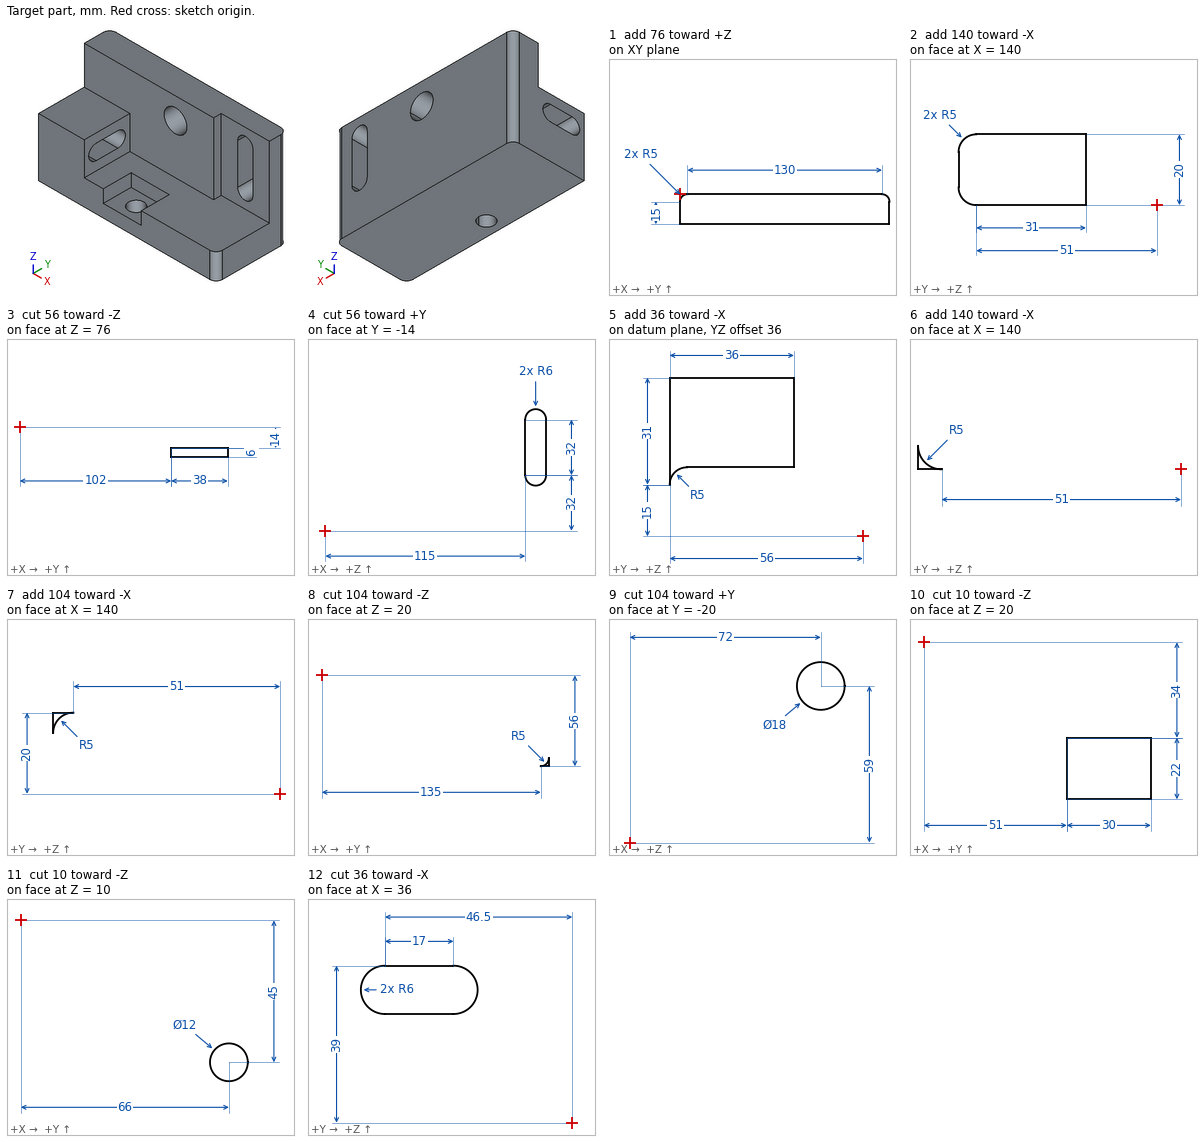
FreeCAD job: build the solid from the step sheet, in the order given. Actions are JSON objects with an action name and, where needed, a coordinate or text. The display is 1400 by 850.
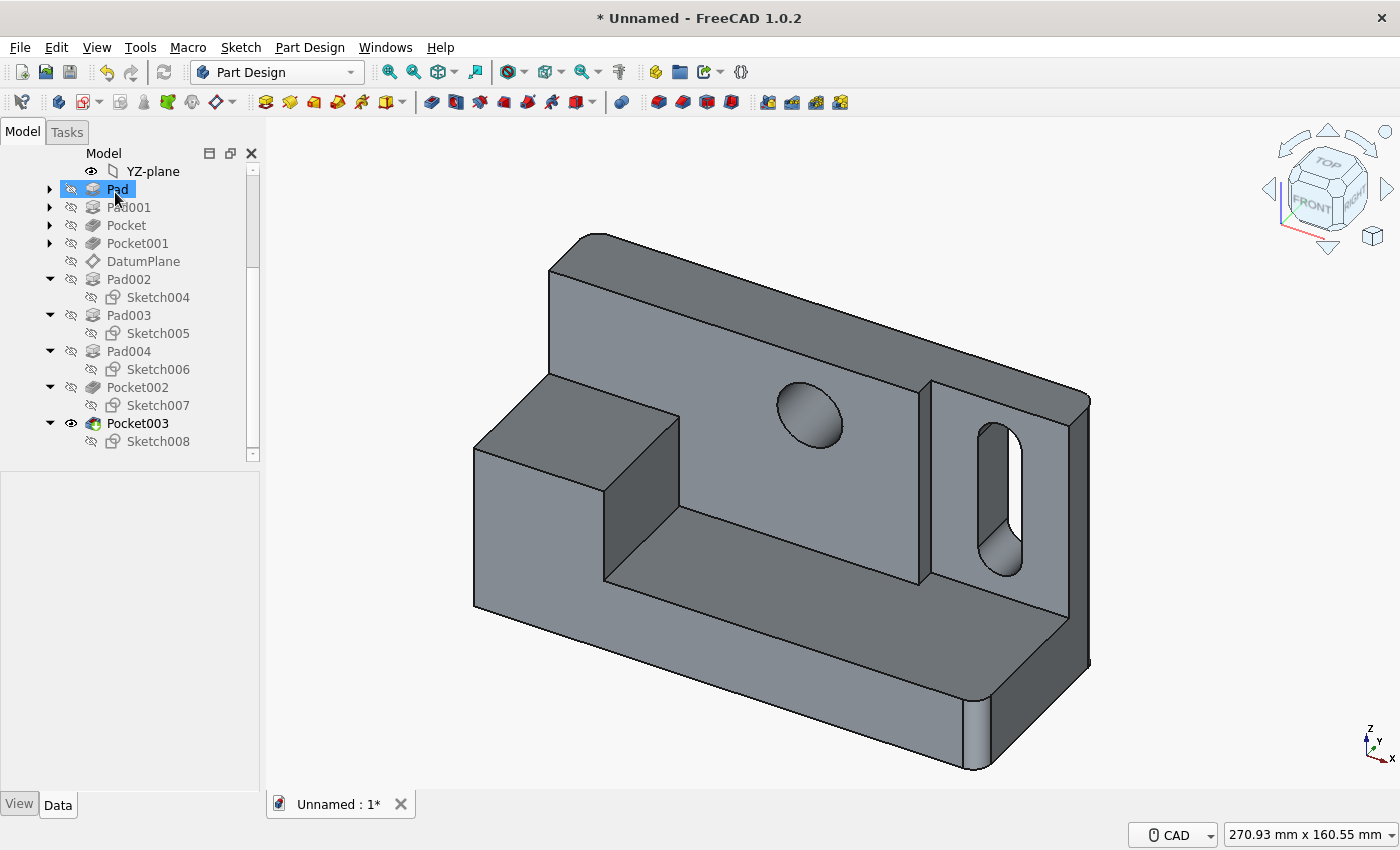
{"action": "left_click", "coordinate": [944, 634]}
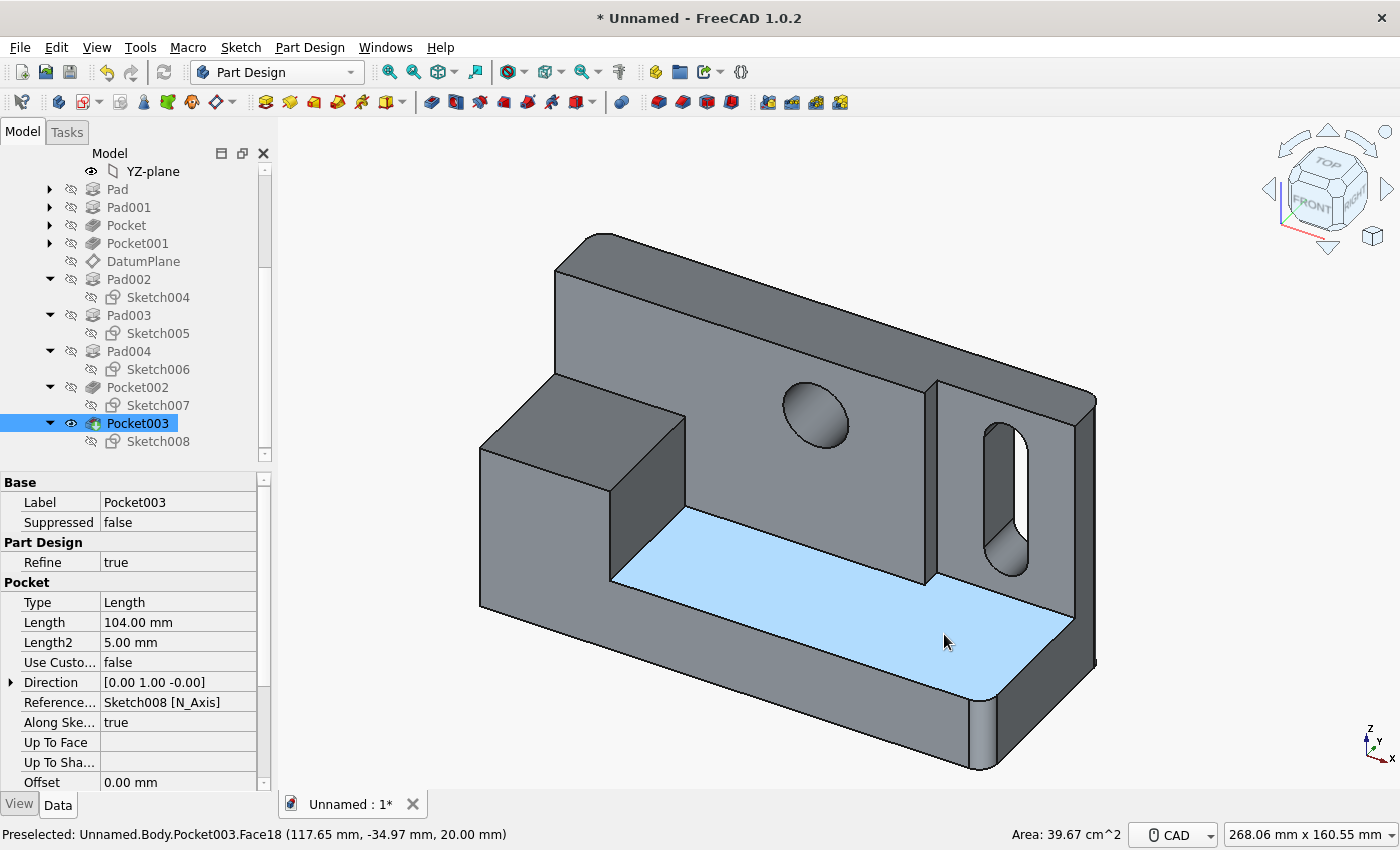
{"action": "left_click", "coordinate": [84, 102]}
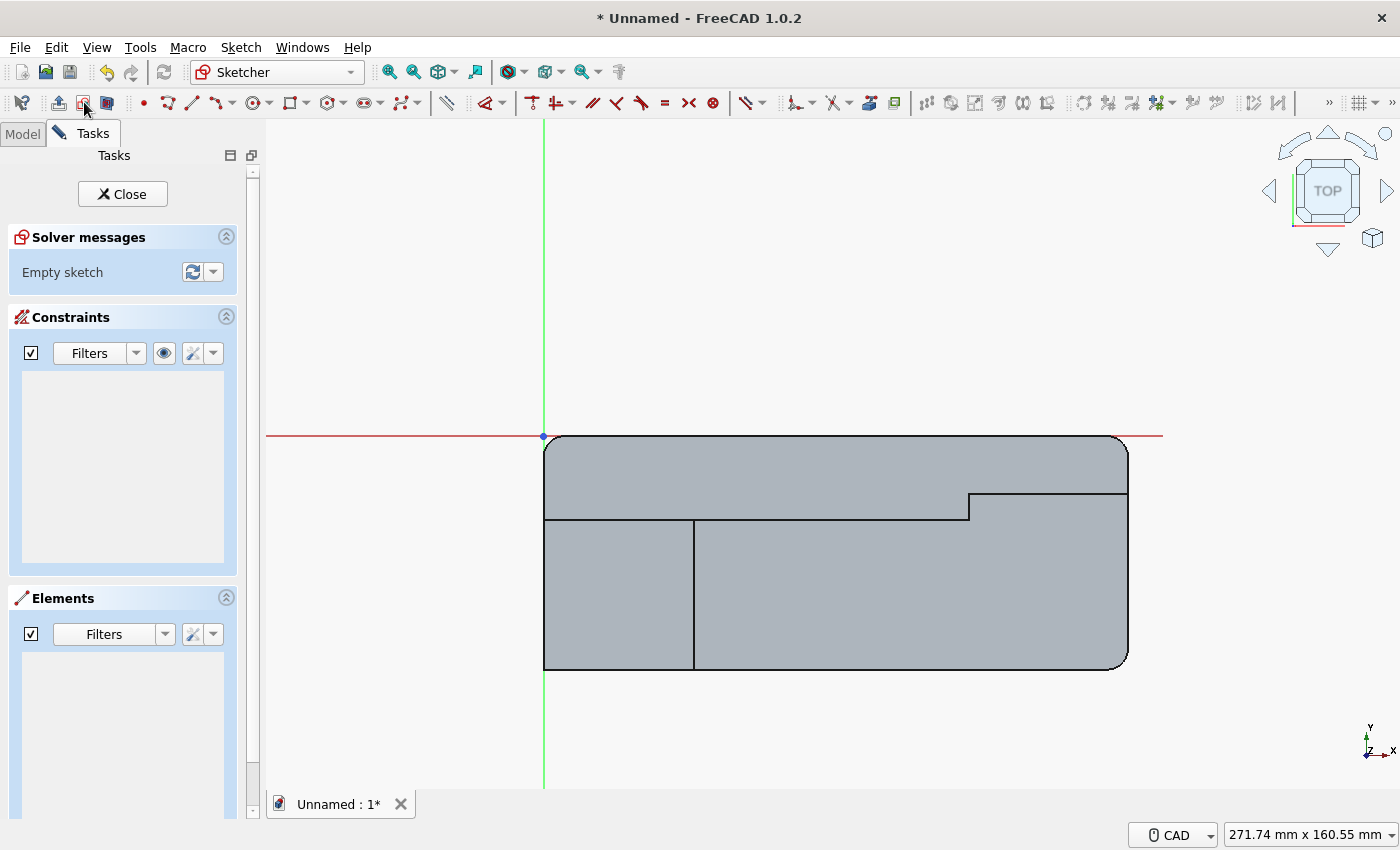
{"action": "key", "text": "q s"}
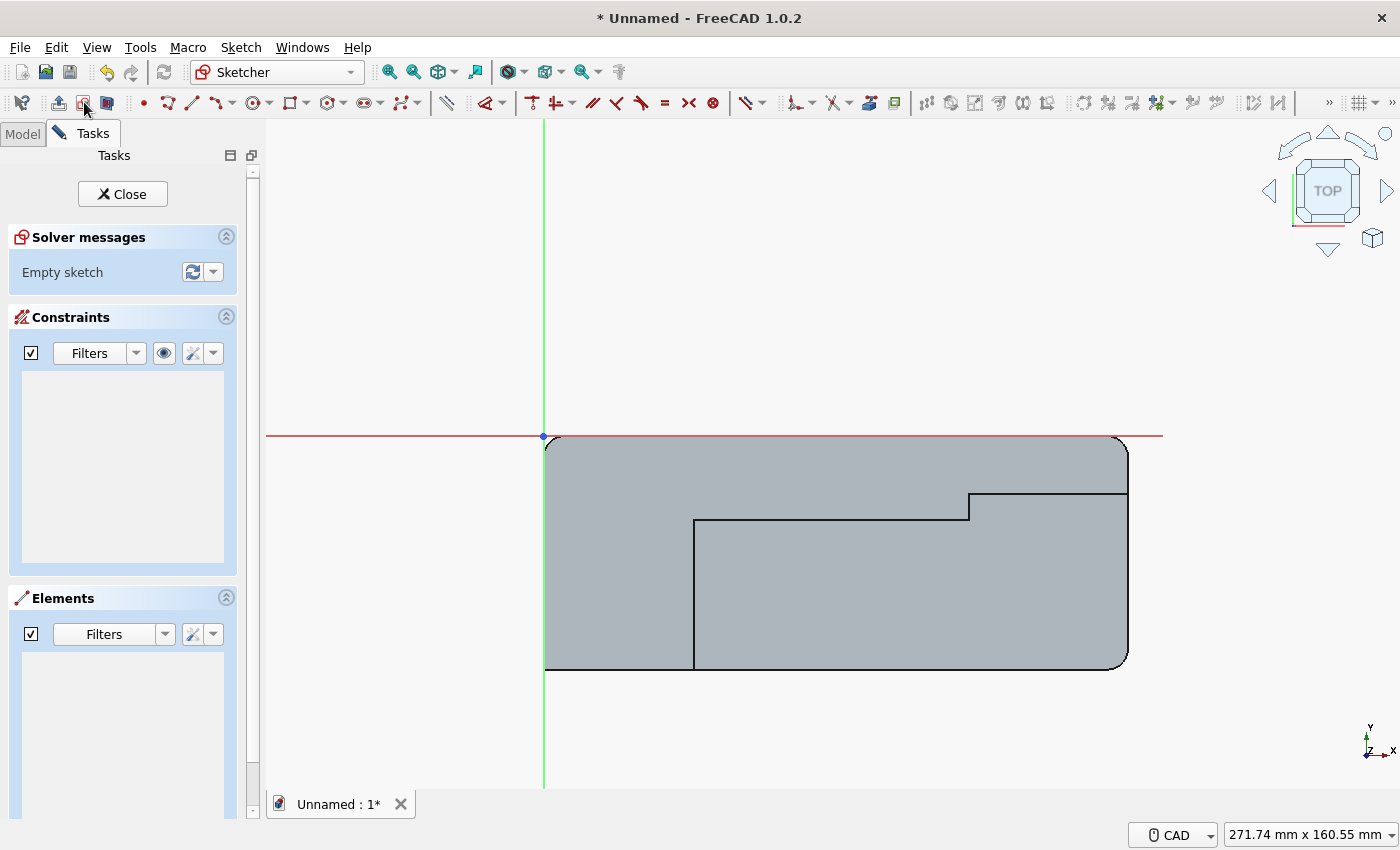
{"action": "scroll", "coordinate": [833, 667], "scroll_direction": "up", "scroll_amount": 8}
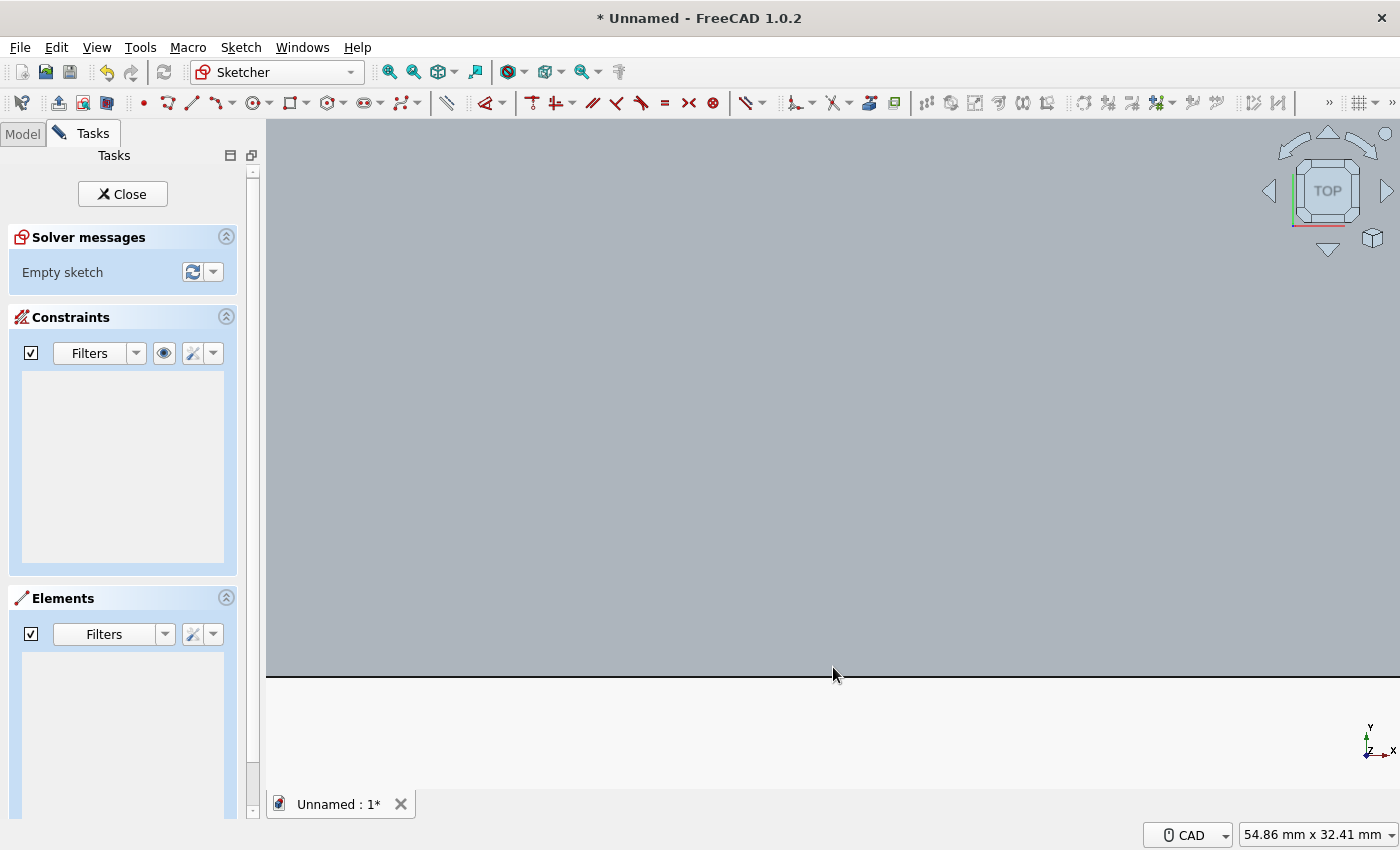
{"action": "left_click", "coordinate": [290, 104]}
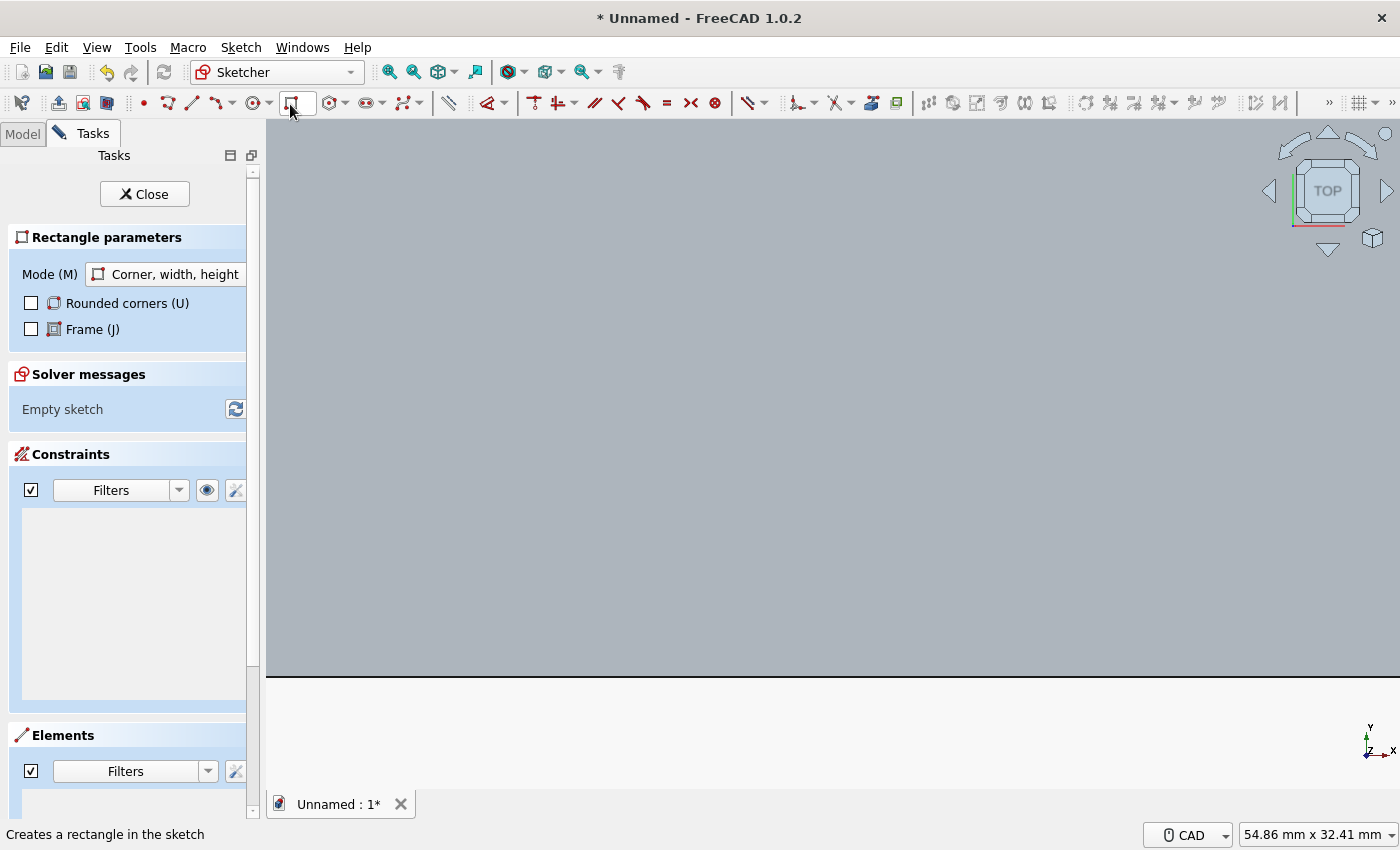
{"action": "left_click", "coordinate": [452, 223]}
{"action": "left_click", "coordinate": [1072, 677]}
{"action": "key", "text": "Escape"}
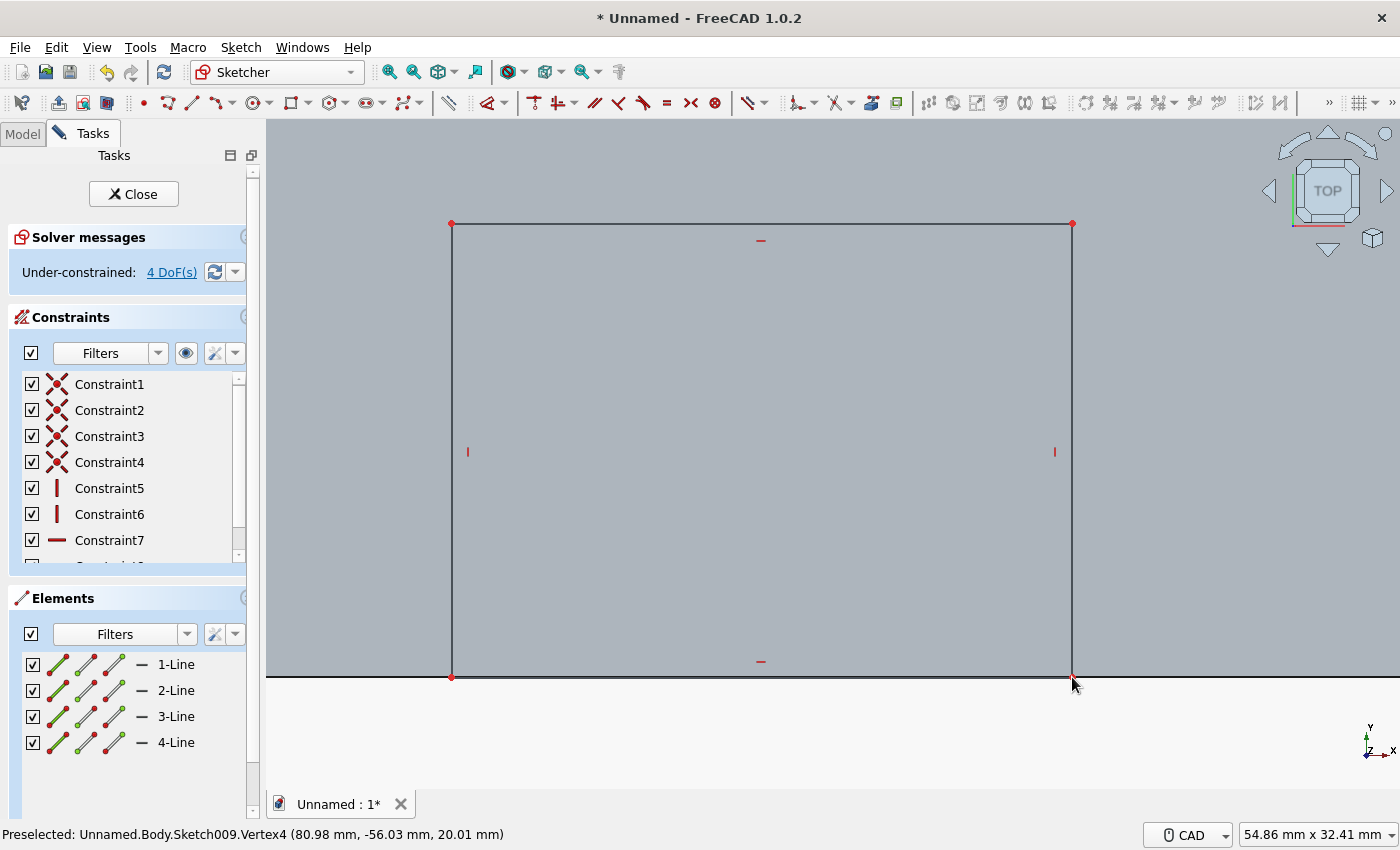
{"action": "key", "text": "d"}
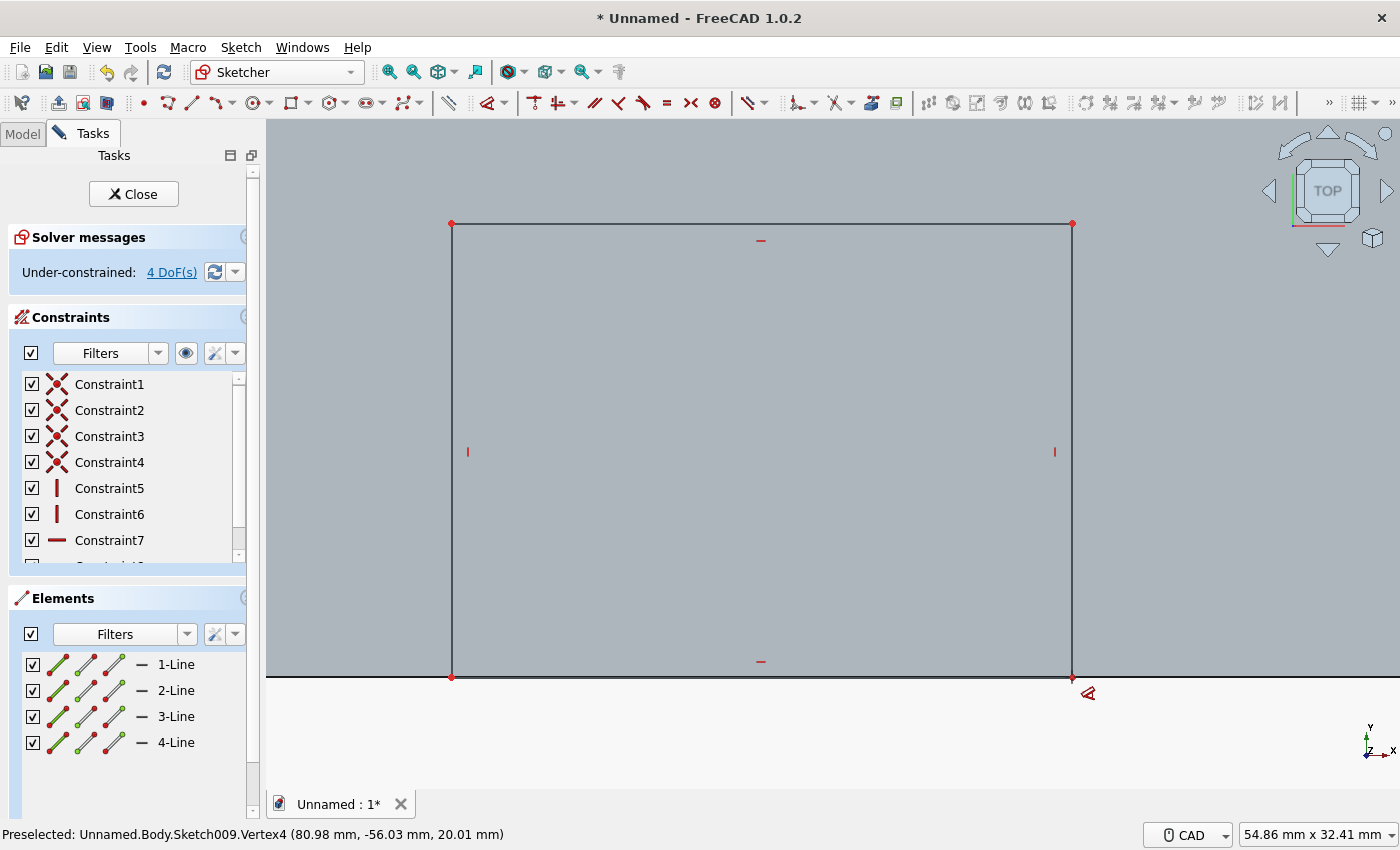
{"action": "left_click", "coordinate": [452, 360]}
{"action": "left_click", "coordinate": [418, 451]}